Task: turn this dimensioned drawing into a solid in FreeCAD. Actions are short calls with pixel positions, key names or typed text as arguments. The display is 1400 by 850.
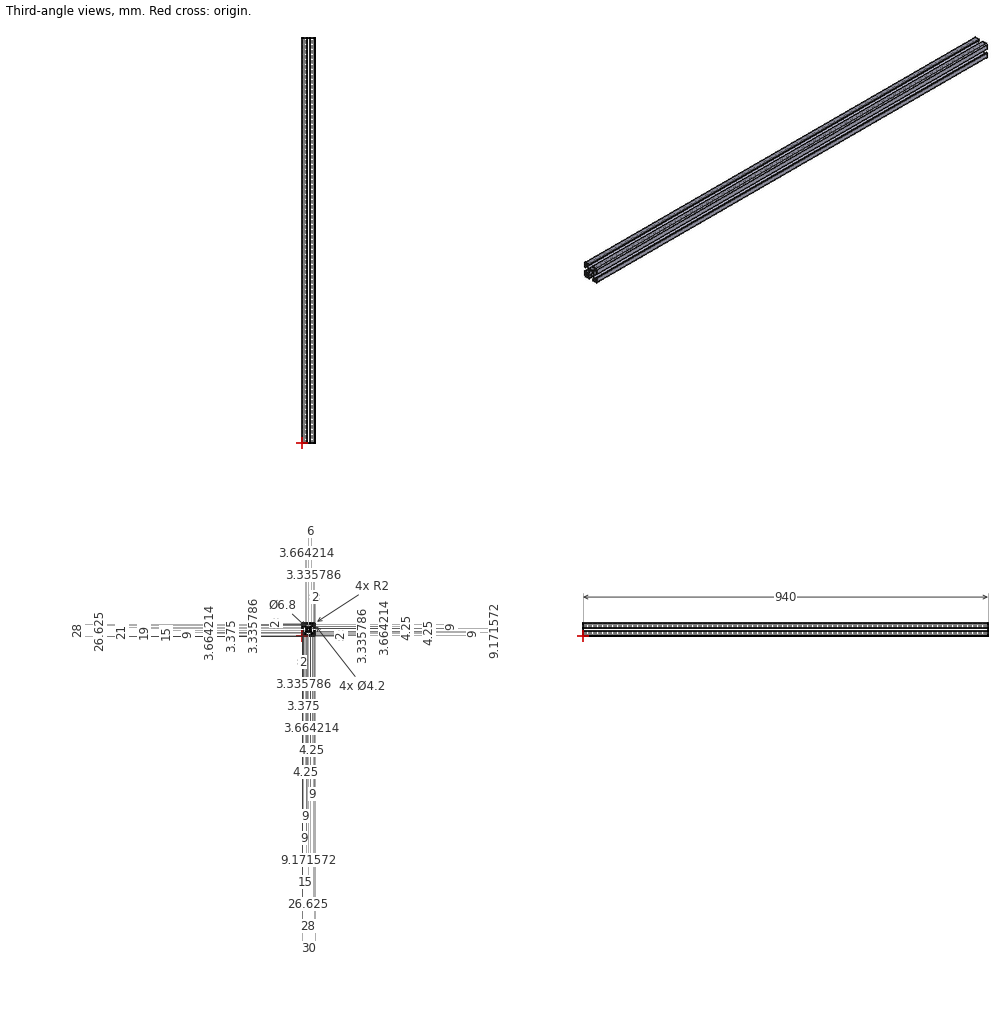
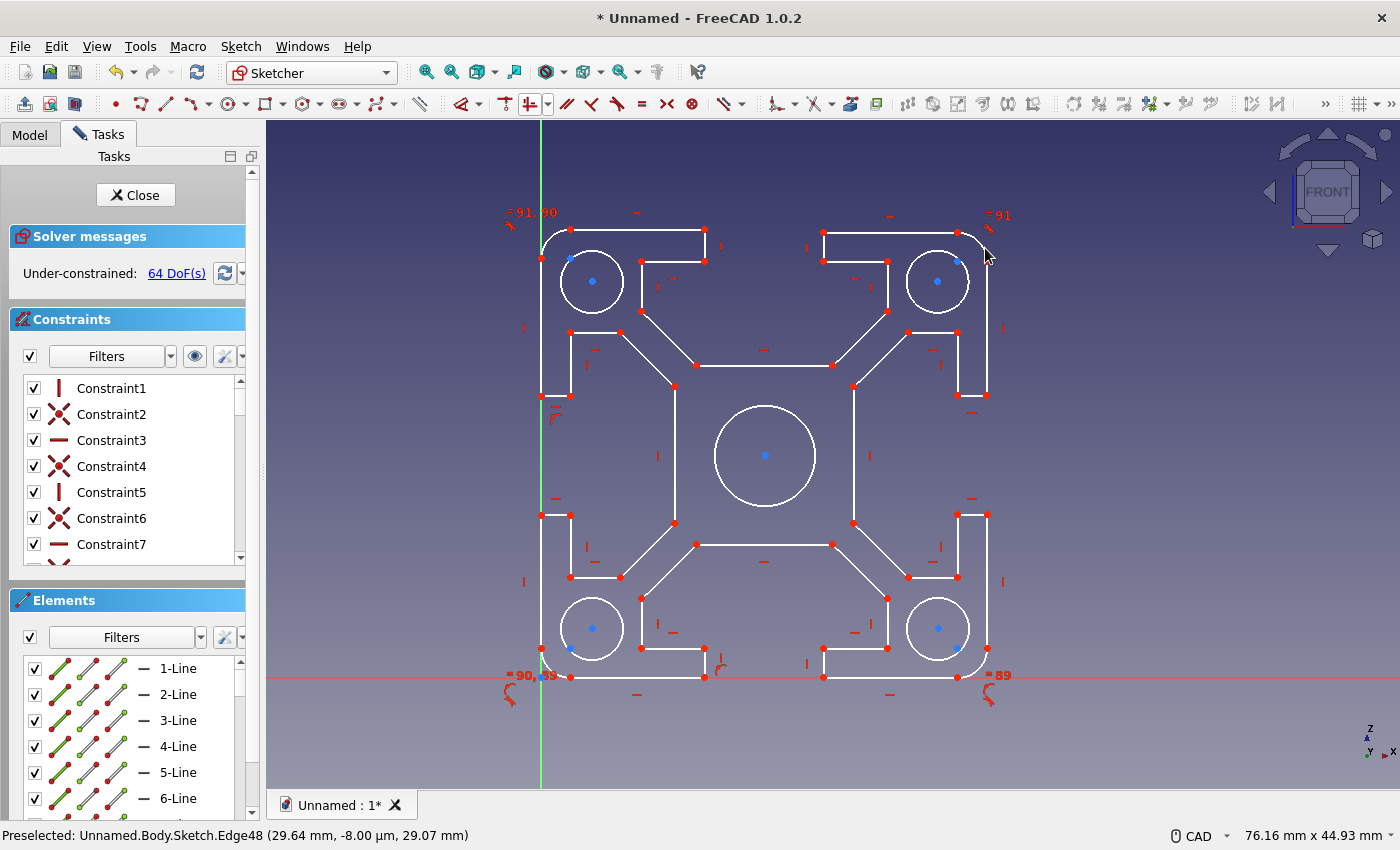
click(916, 260)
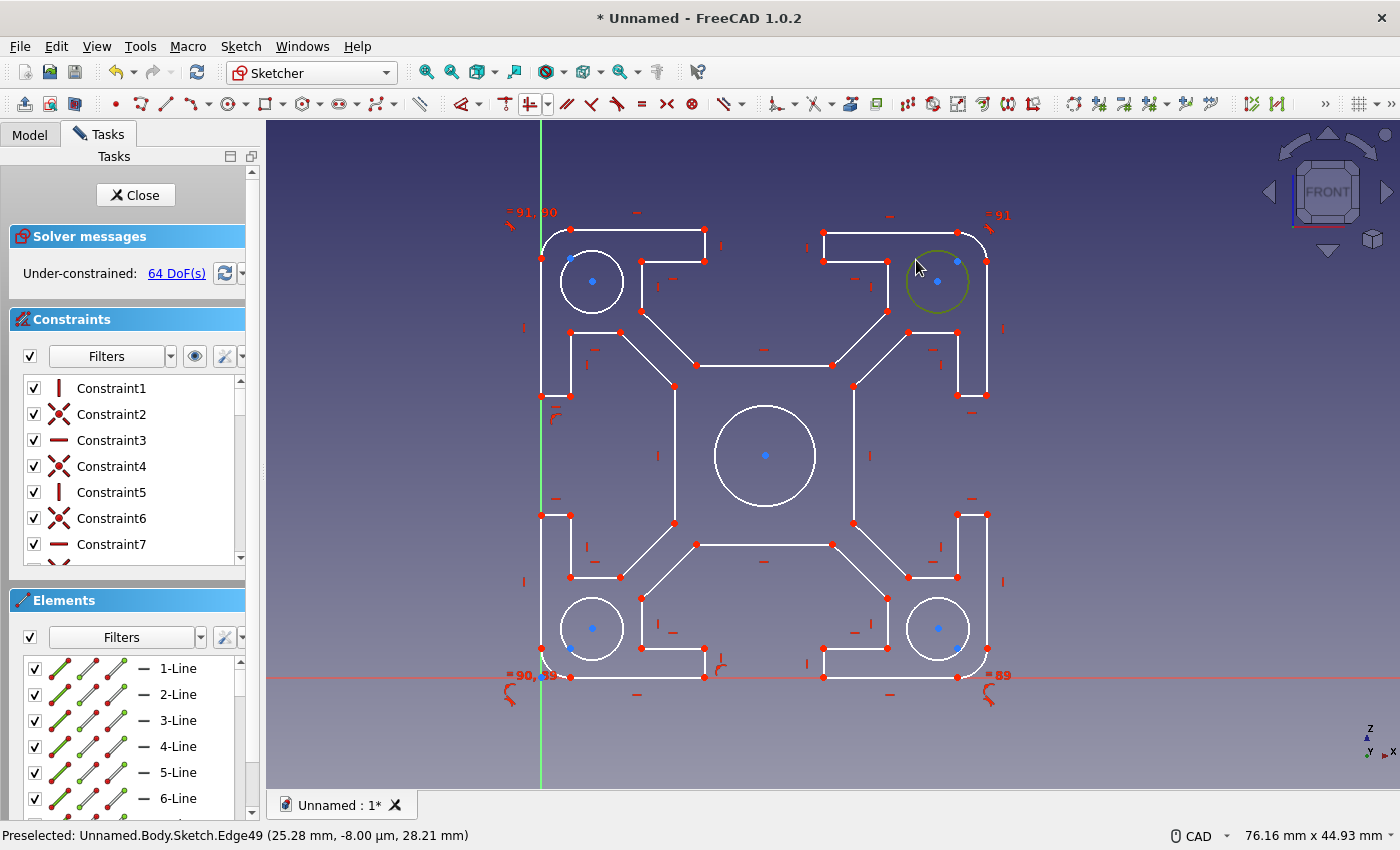
click(614, 260)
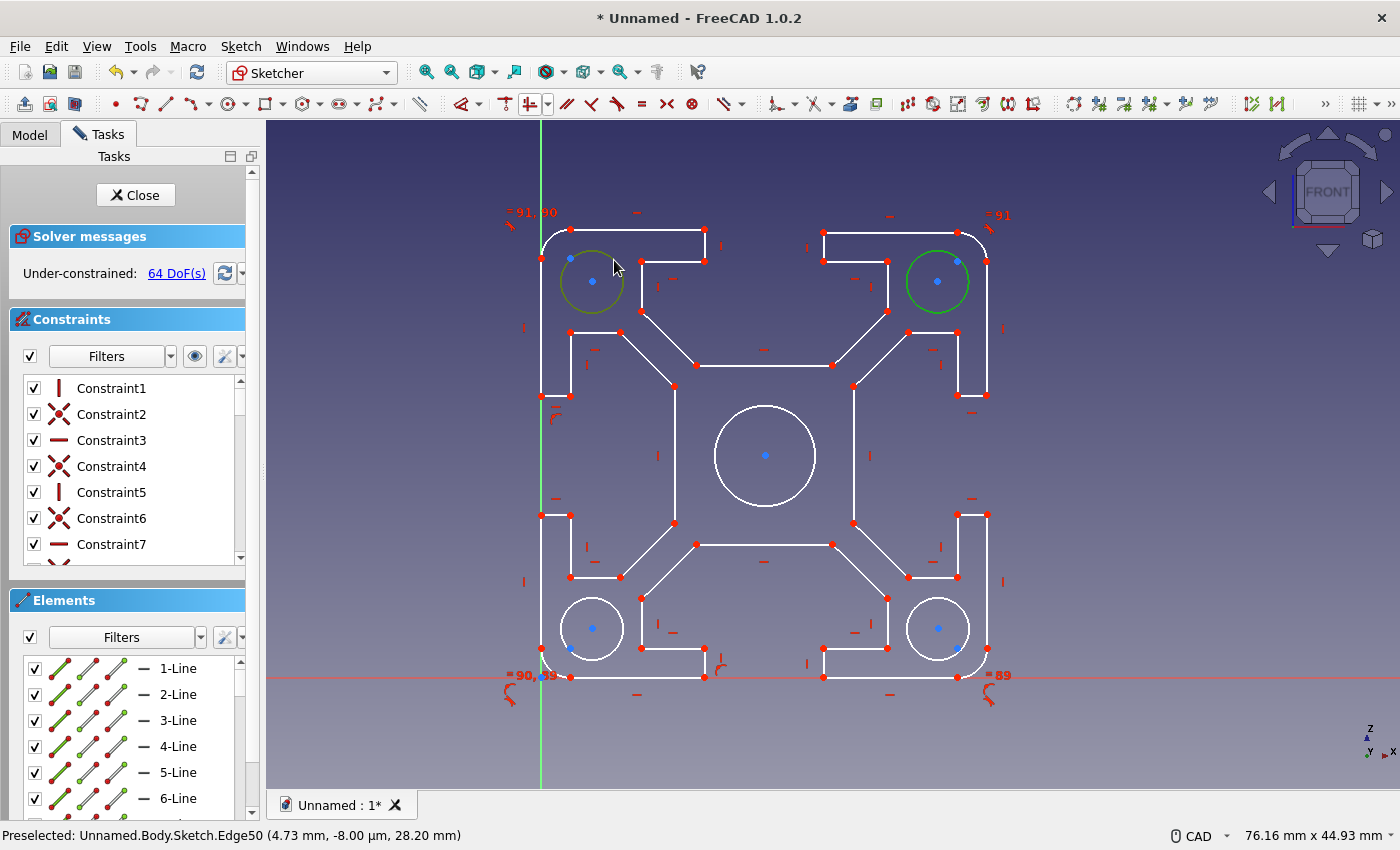
click(960, 607)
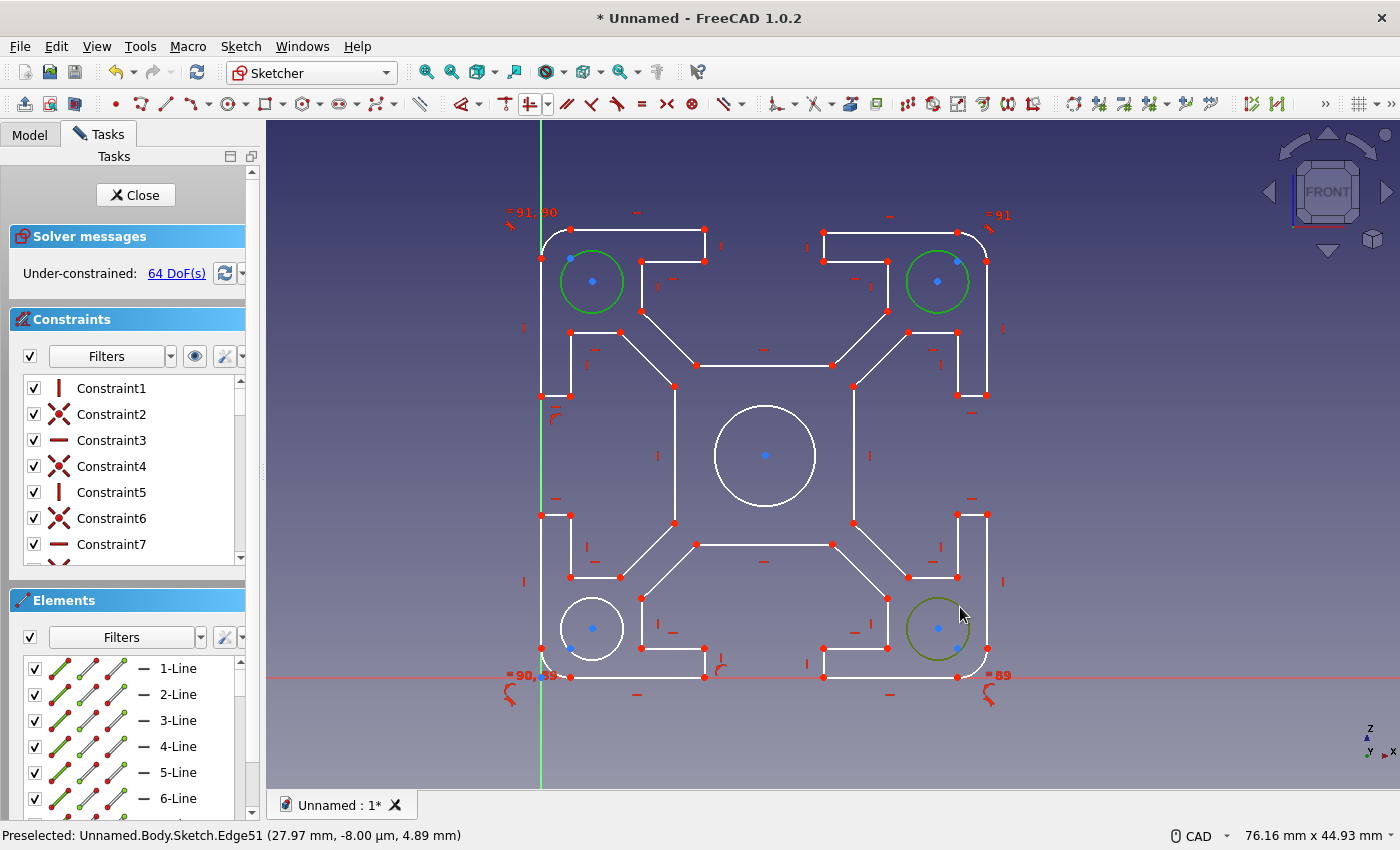
click(614, 607)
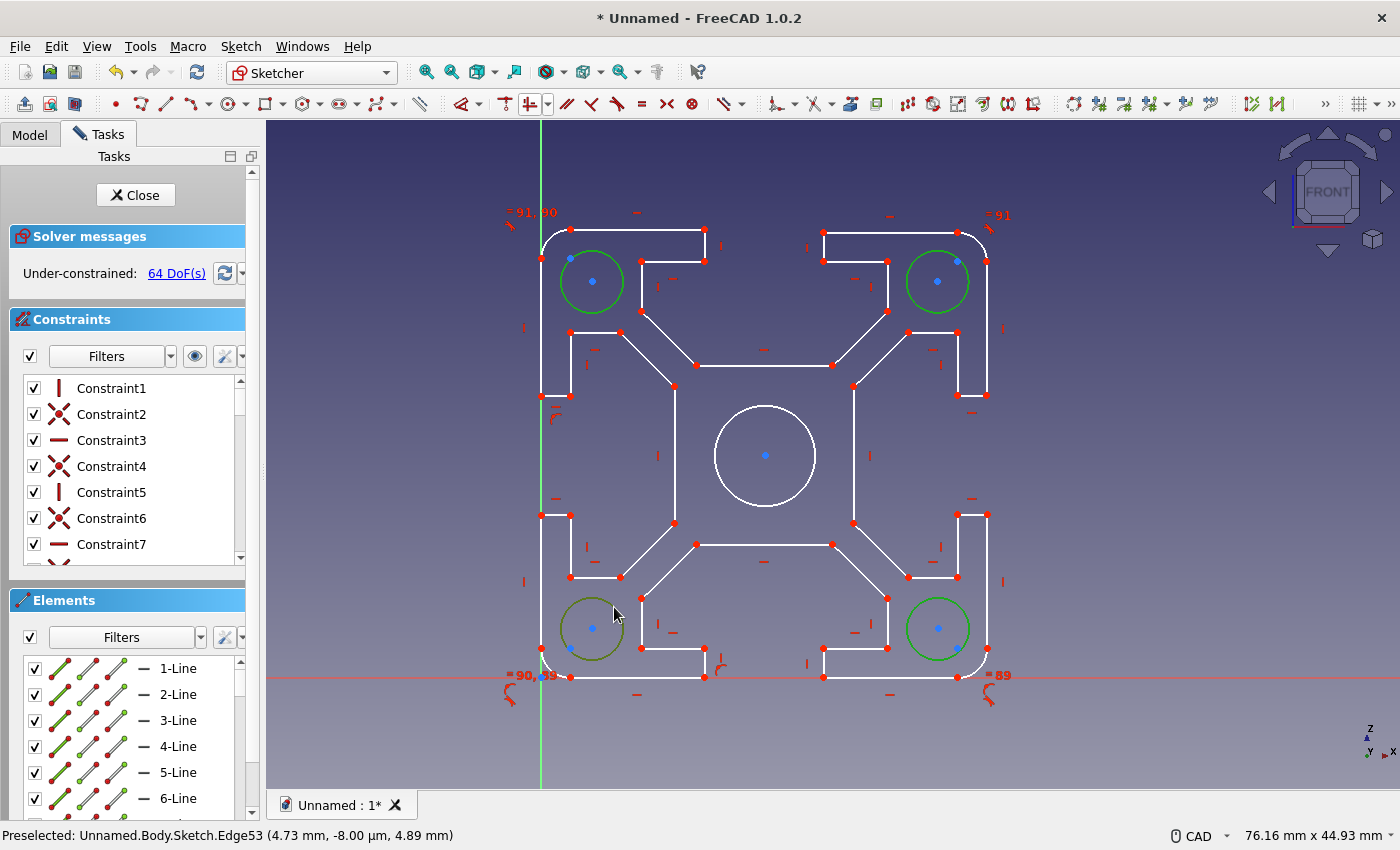
key(e)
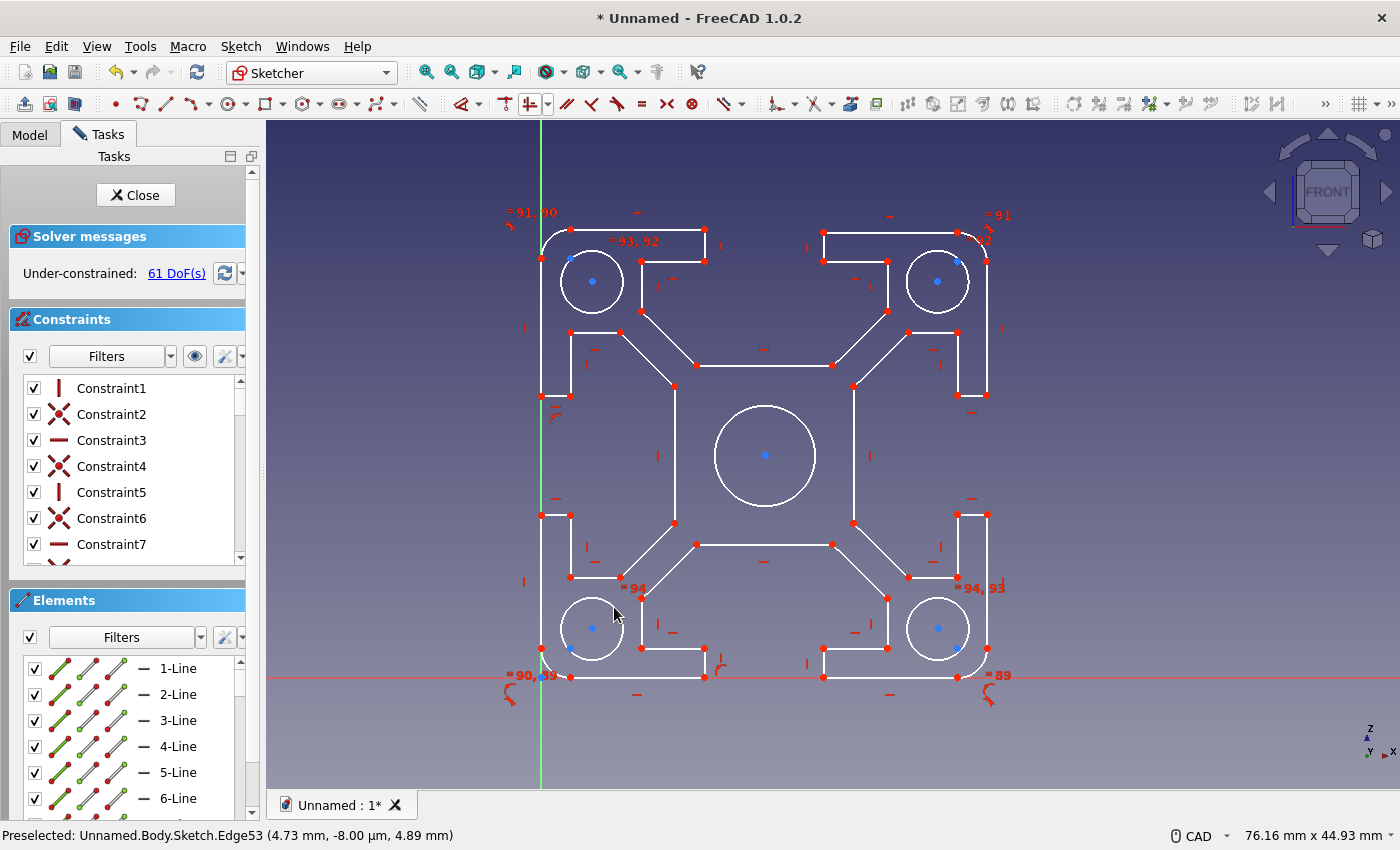
click(460, 104)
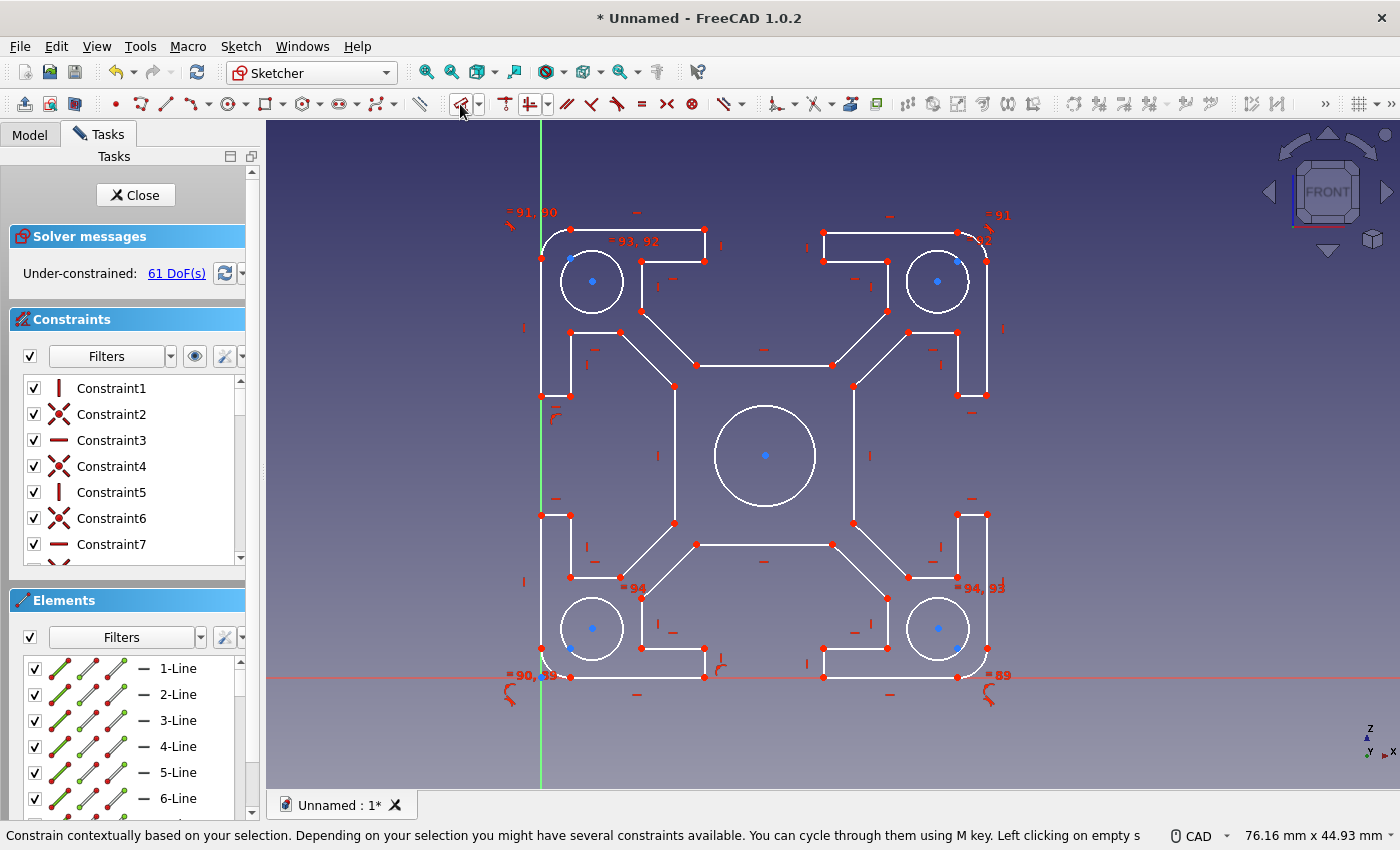
scroll(971, 675, up, 2)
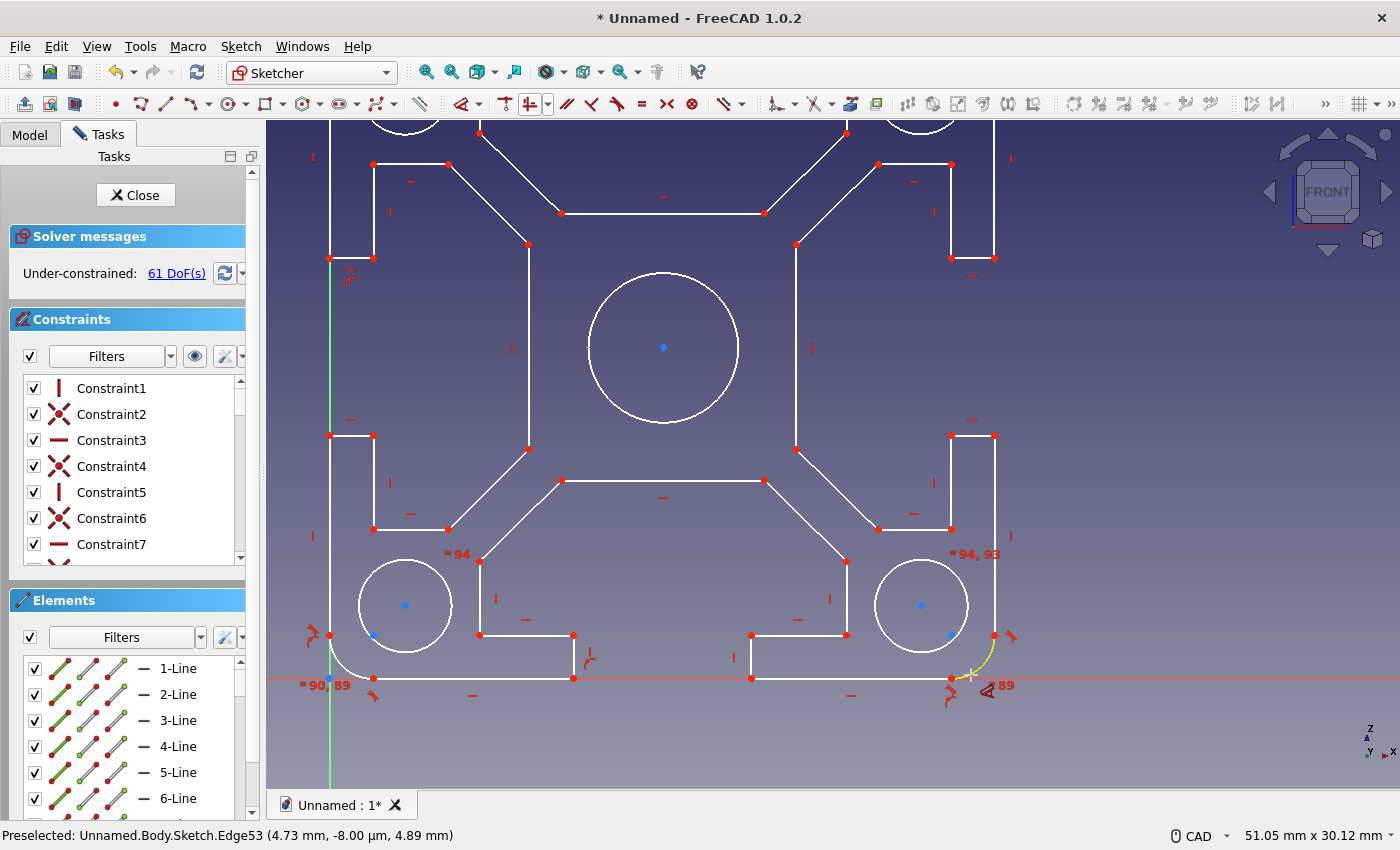
click(971, 674)
click(986, 702)